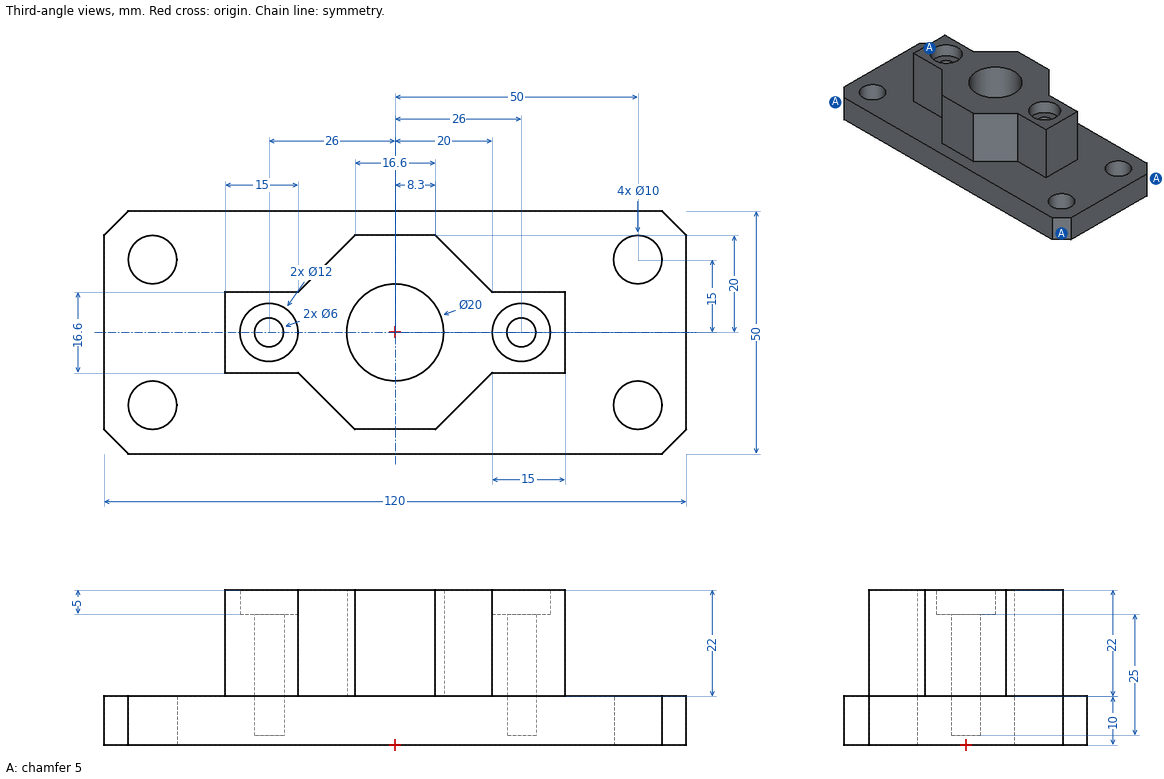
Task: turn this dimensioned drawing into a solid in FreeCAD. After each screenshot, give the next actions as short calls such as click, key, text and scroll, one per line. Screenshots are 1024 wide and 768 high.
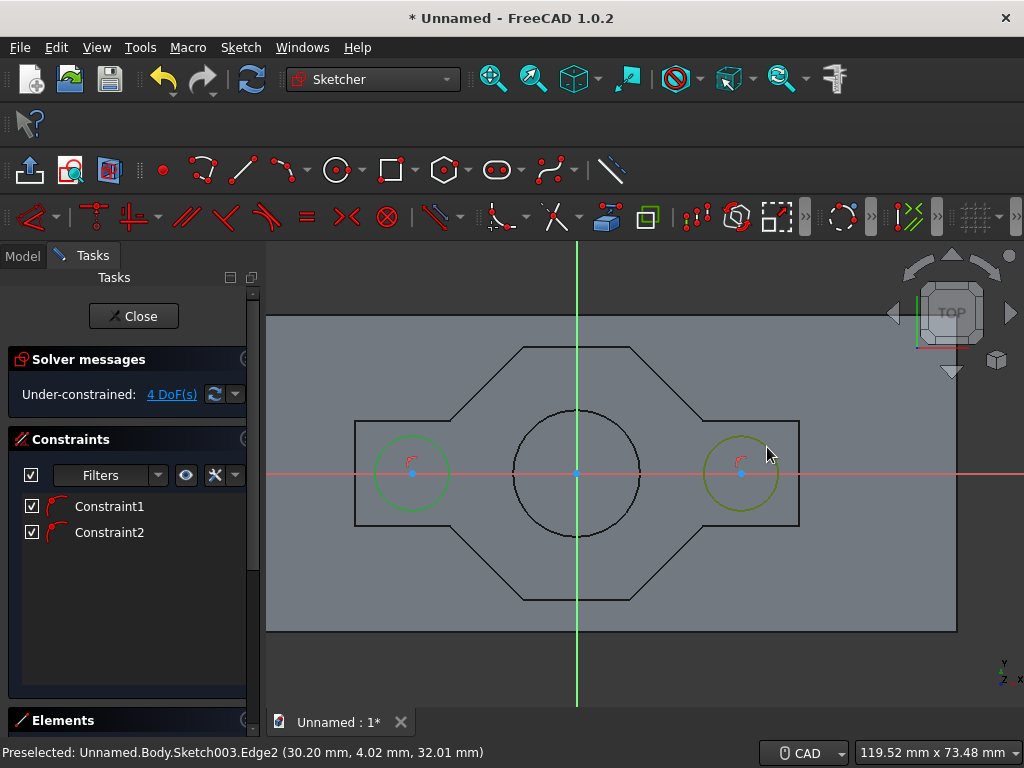
click(308, 218)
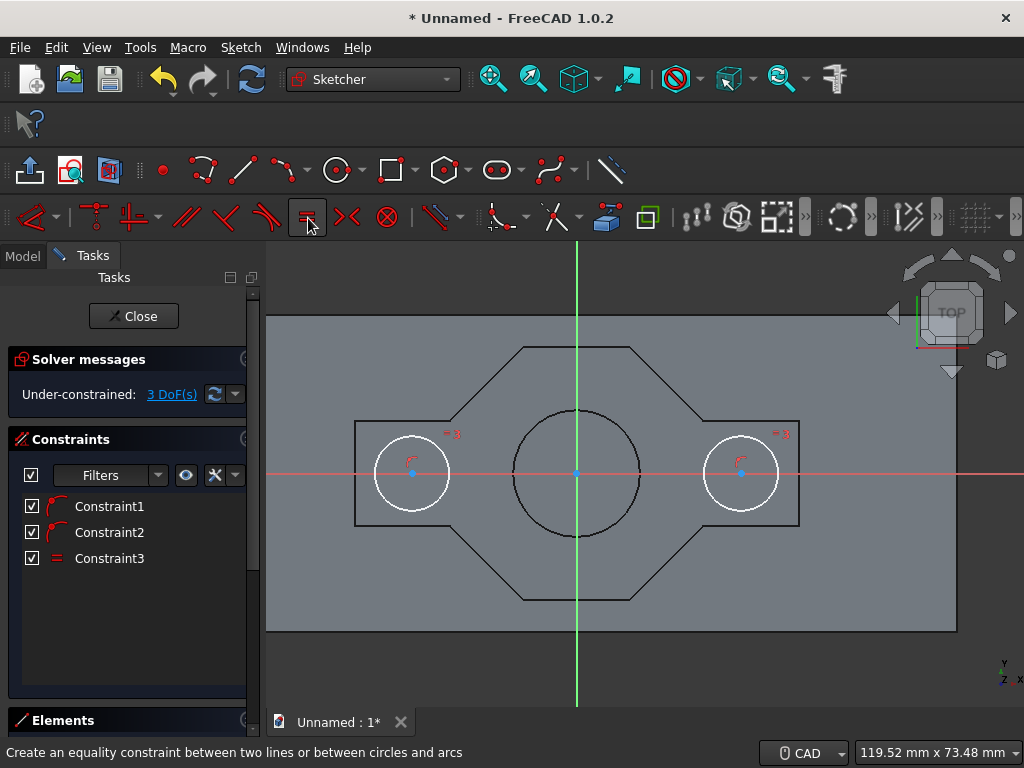
click(32, 218)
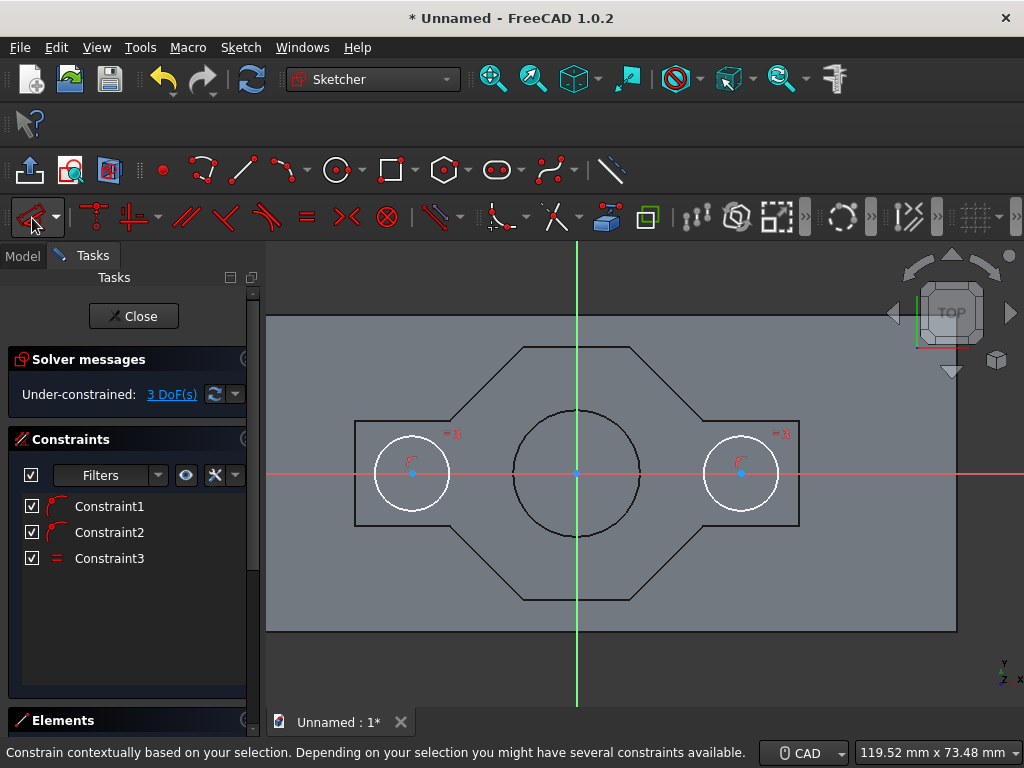
click(438, 447)
click(460, 424)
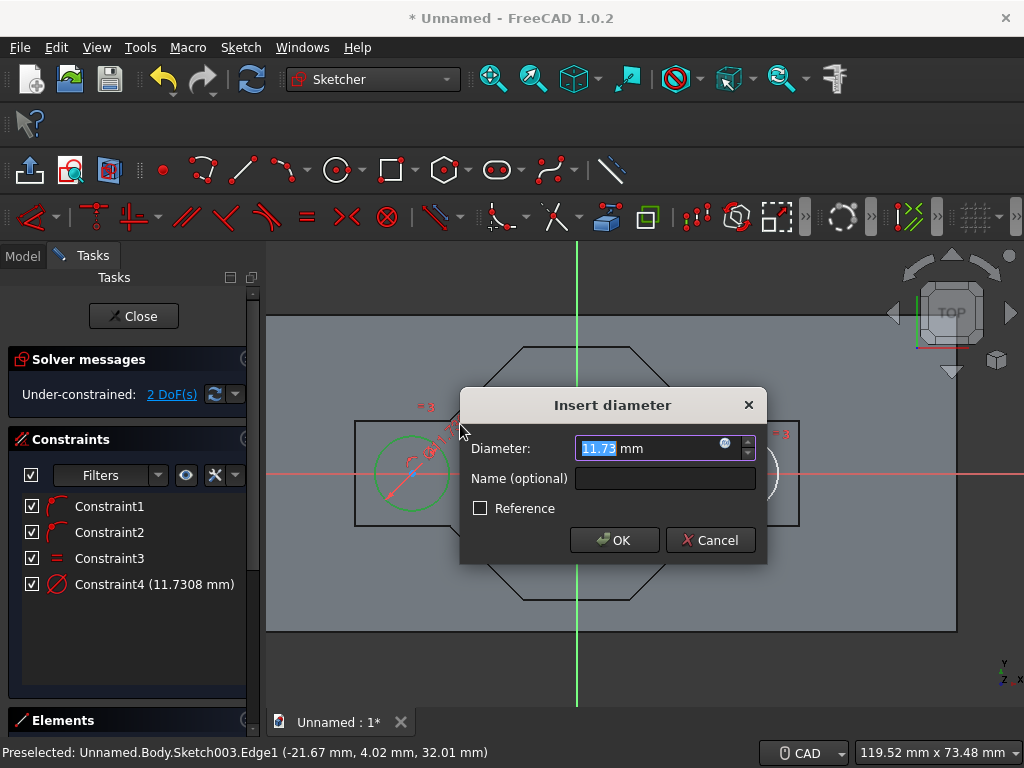
text(12)
key(Return)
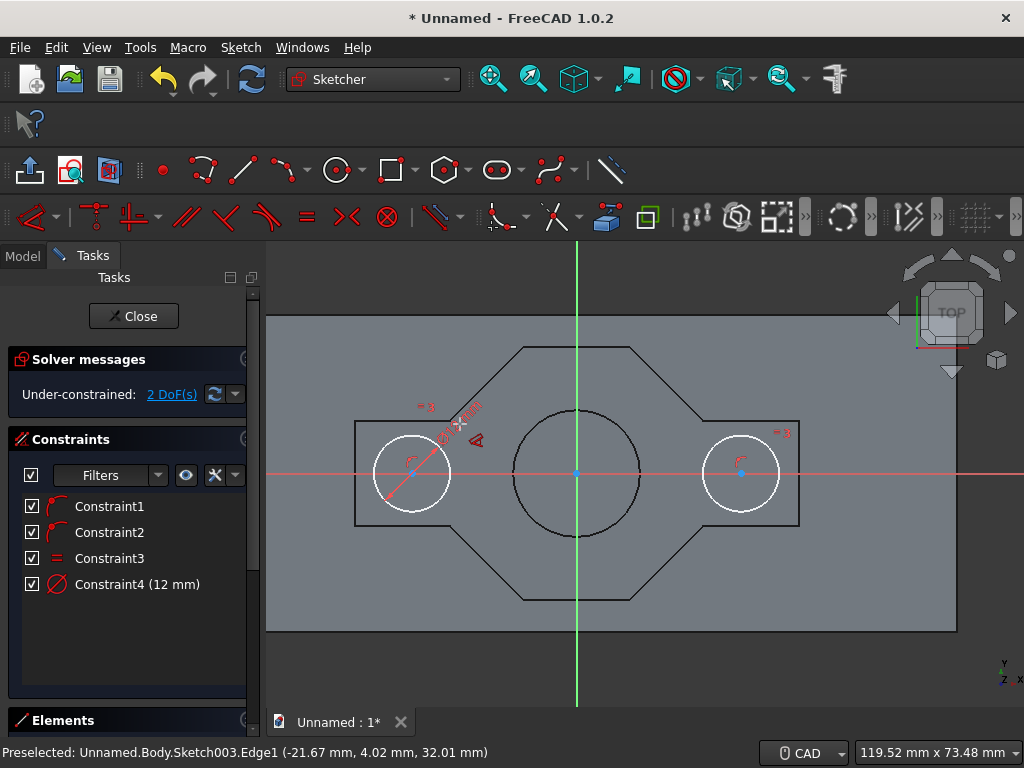
click(412, 474)
click(494, 508)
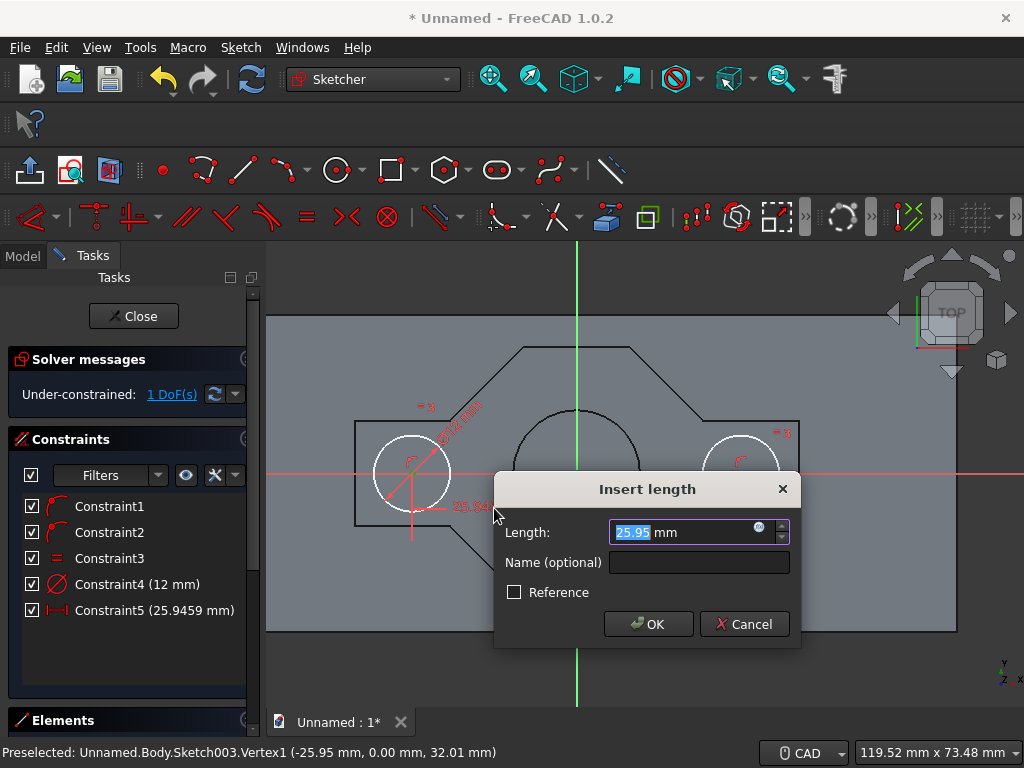
text(26)
key(Return)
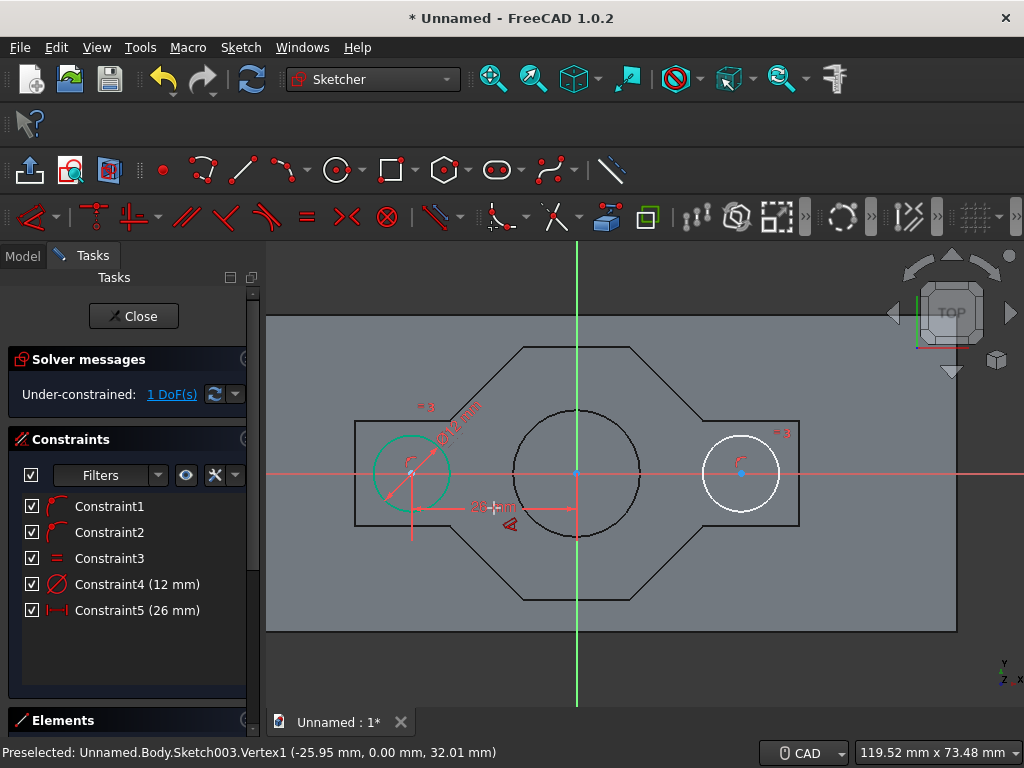
click(741, 474)
click(659, 508)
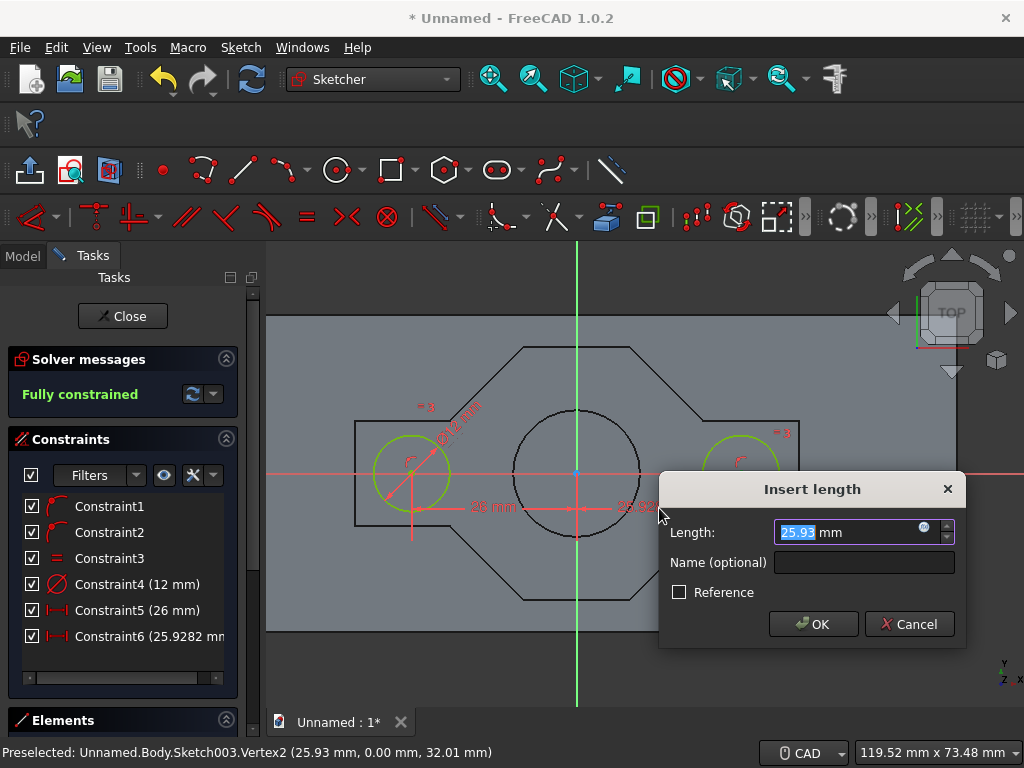
text(26)
key(Return)
key(Escape)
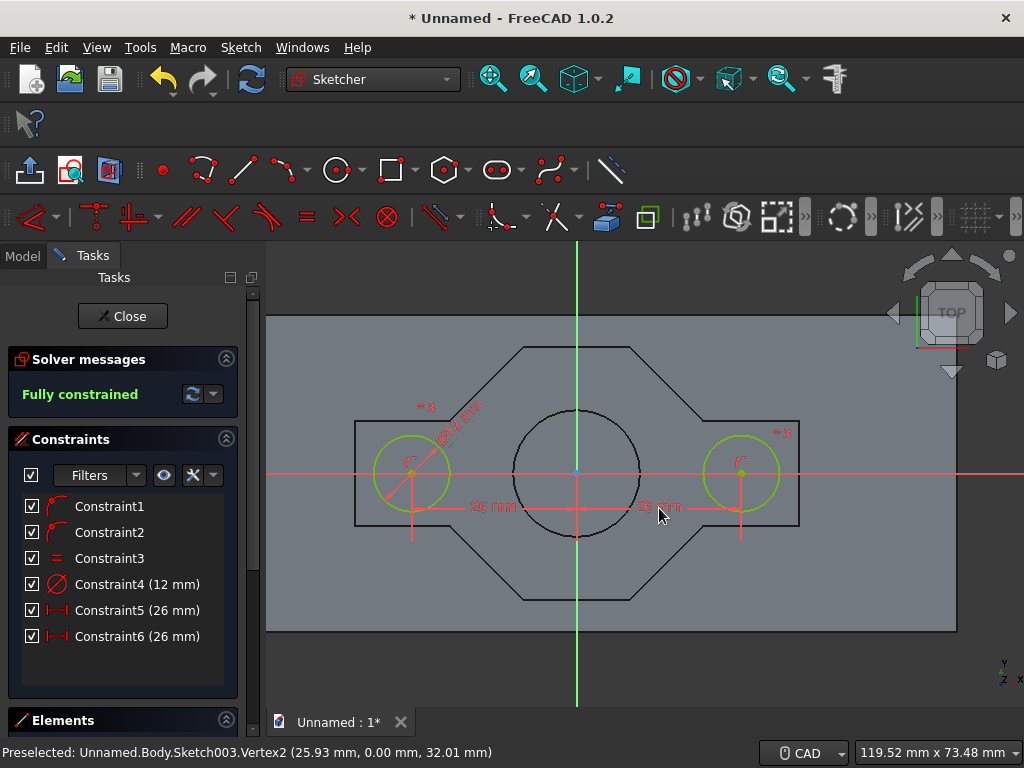
click(123, 316)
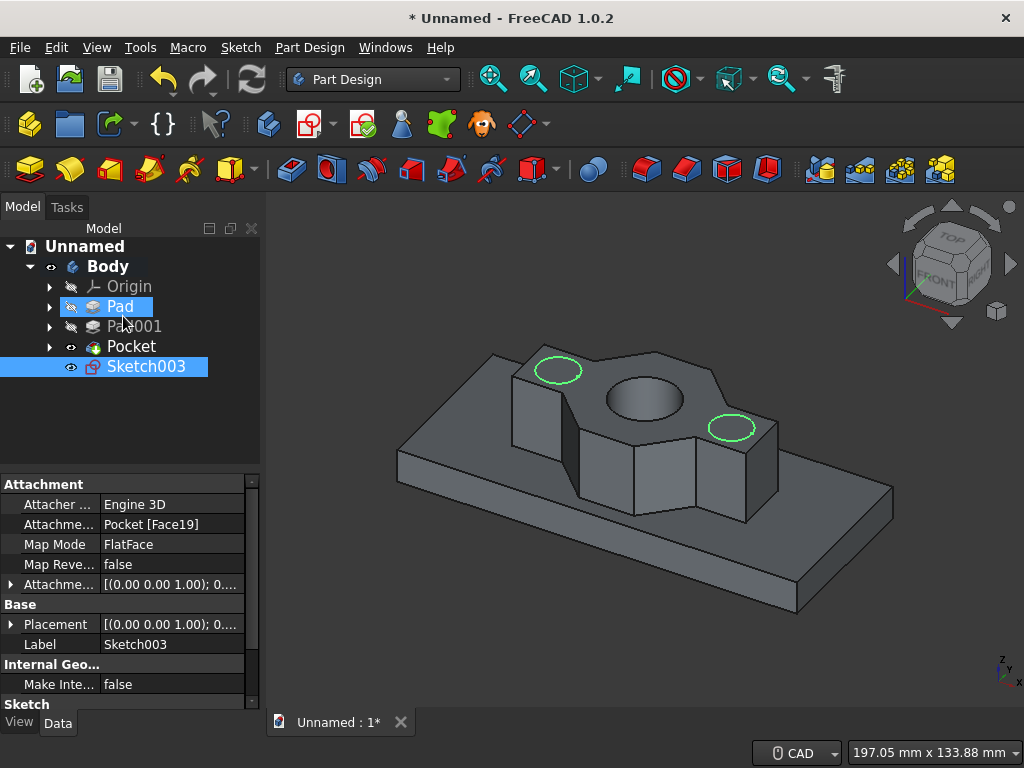
click(292, 170)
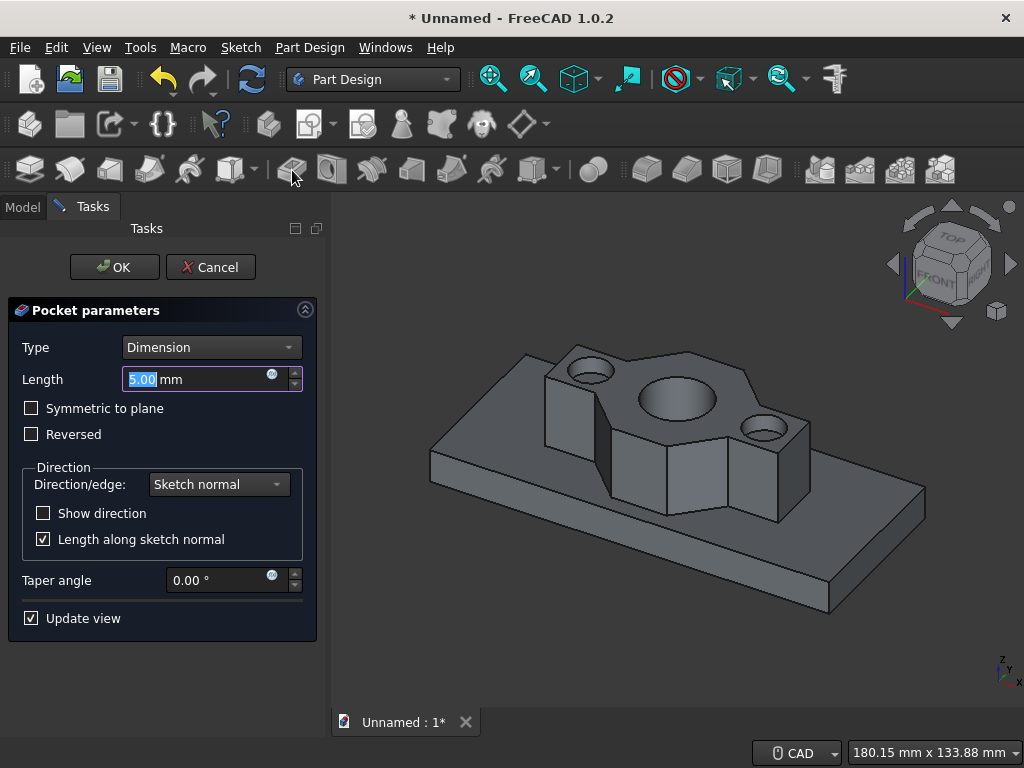
text(5)
key(Tab)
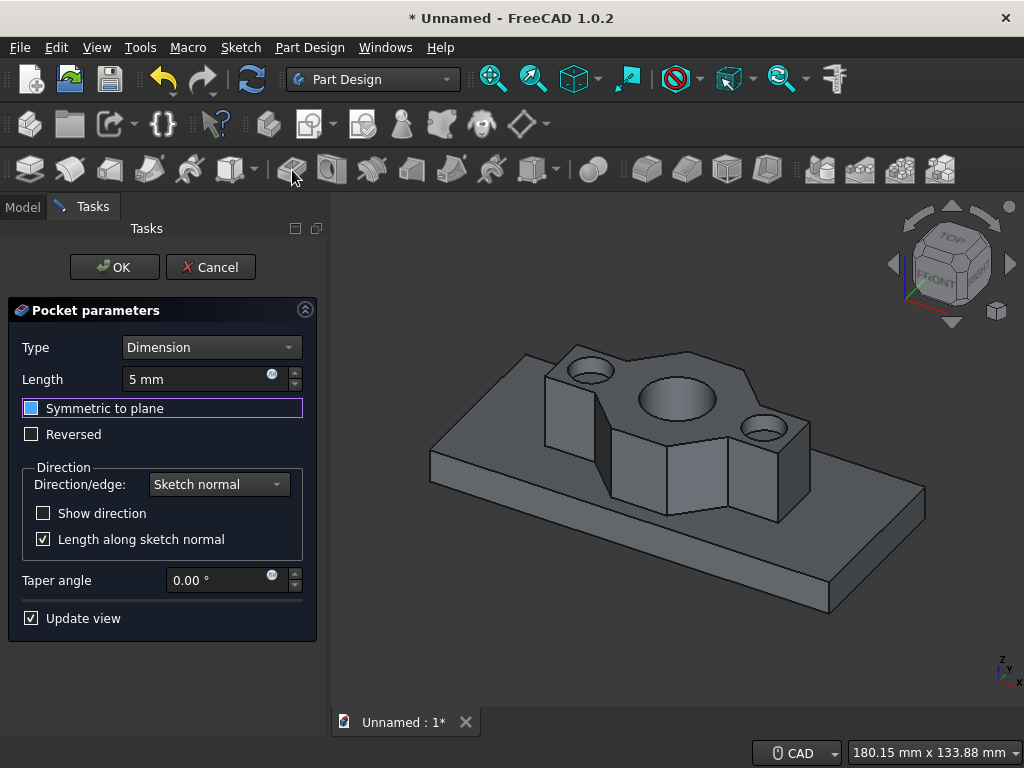
click(115, 267)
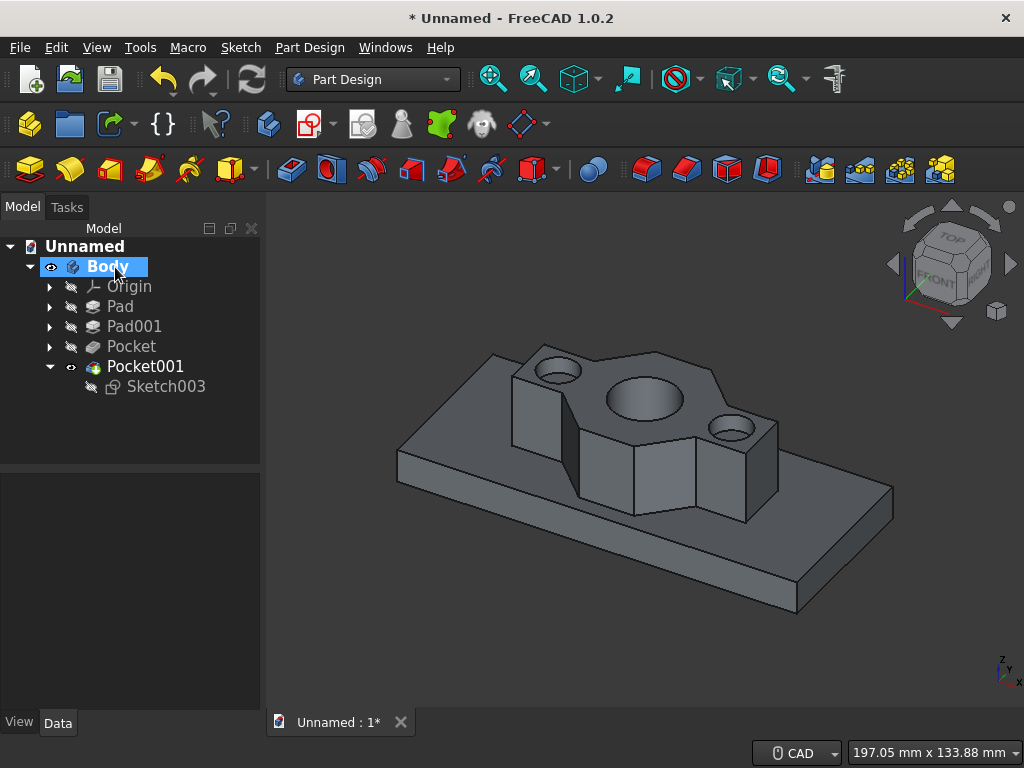
key(0)